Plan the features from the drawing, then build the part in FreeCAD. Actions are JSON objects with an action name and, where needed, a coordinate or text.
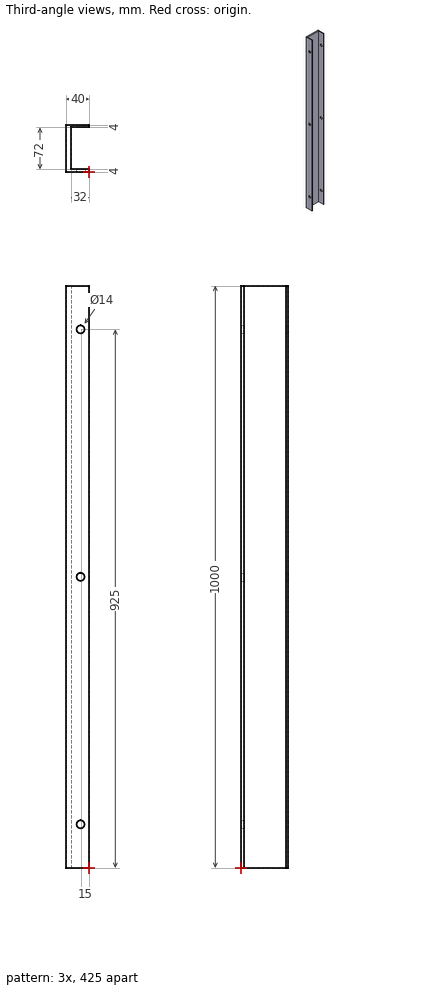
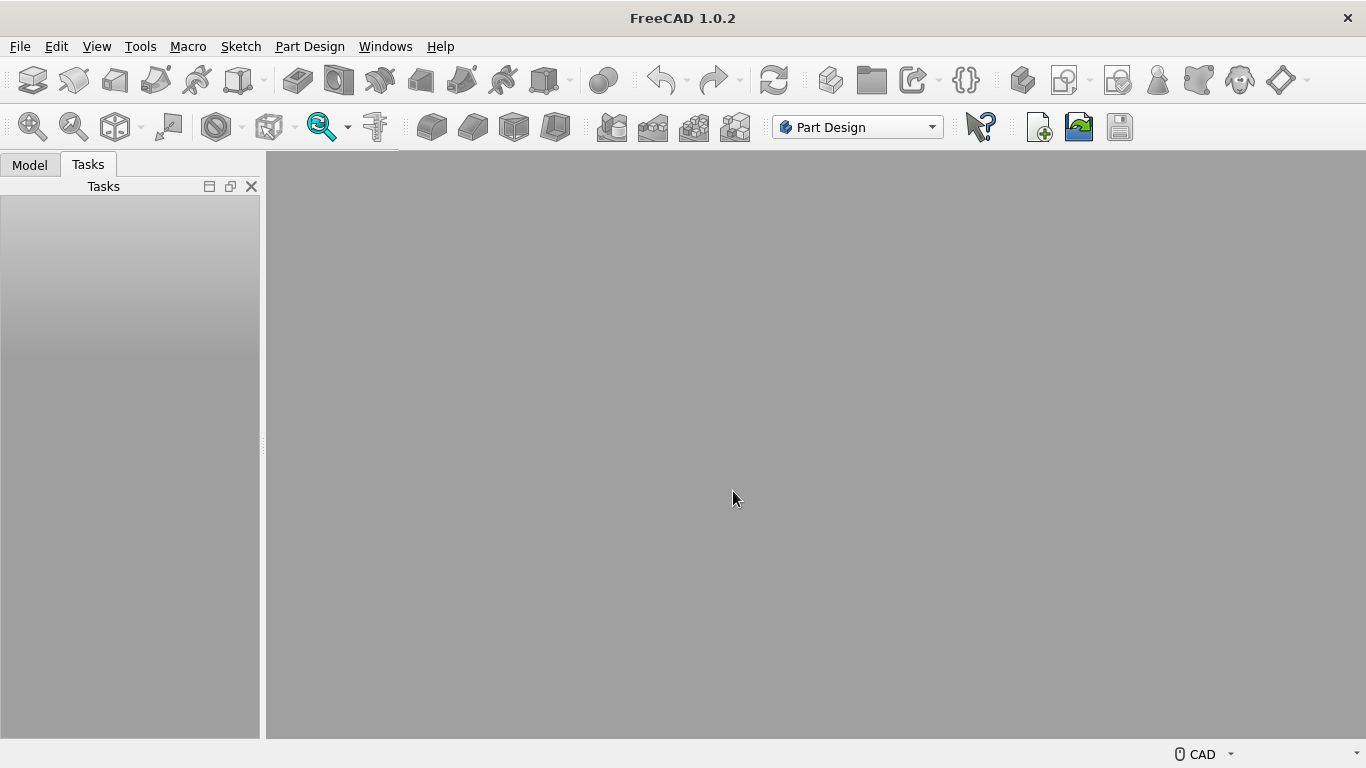
{"action": "left_click", "coordinate": [1038, 128]}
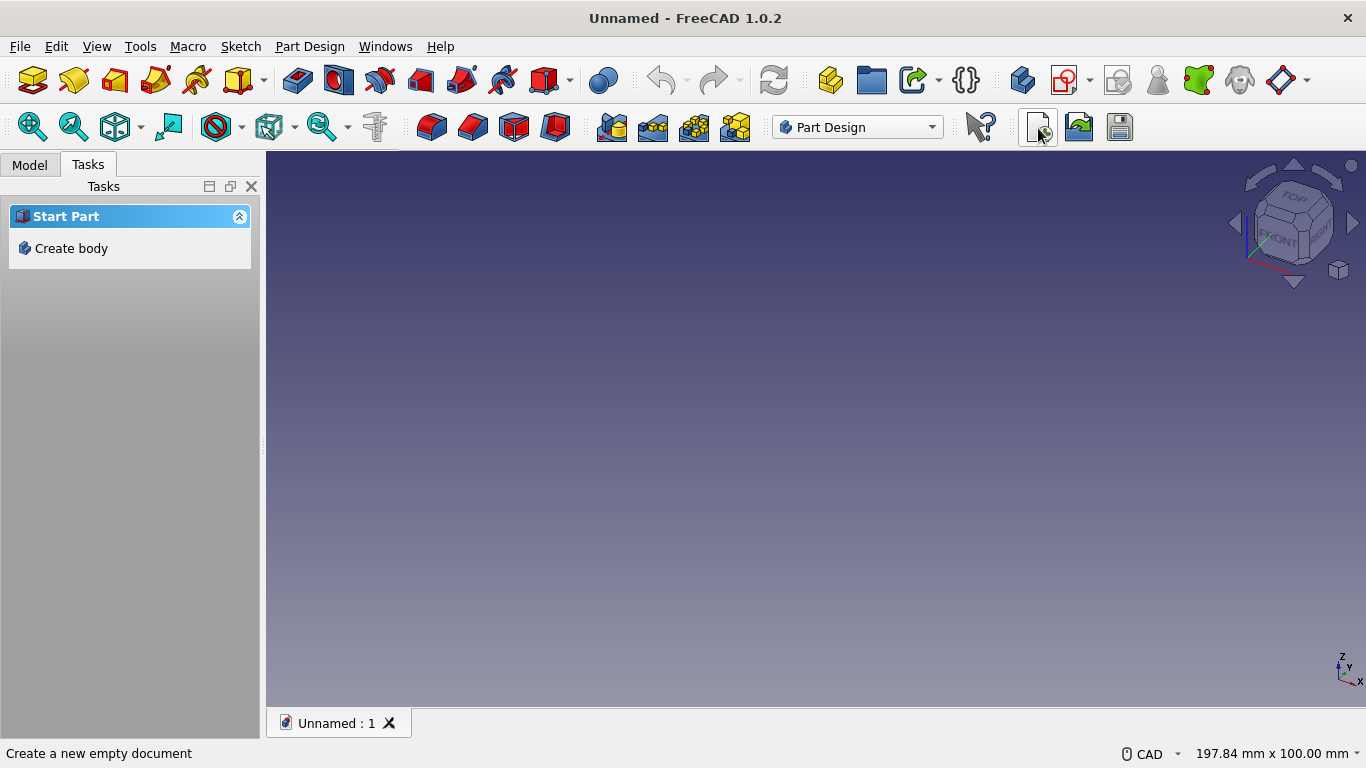
{"action": "left_click", "coordinate": [1064, 80]}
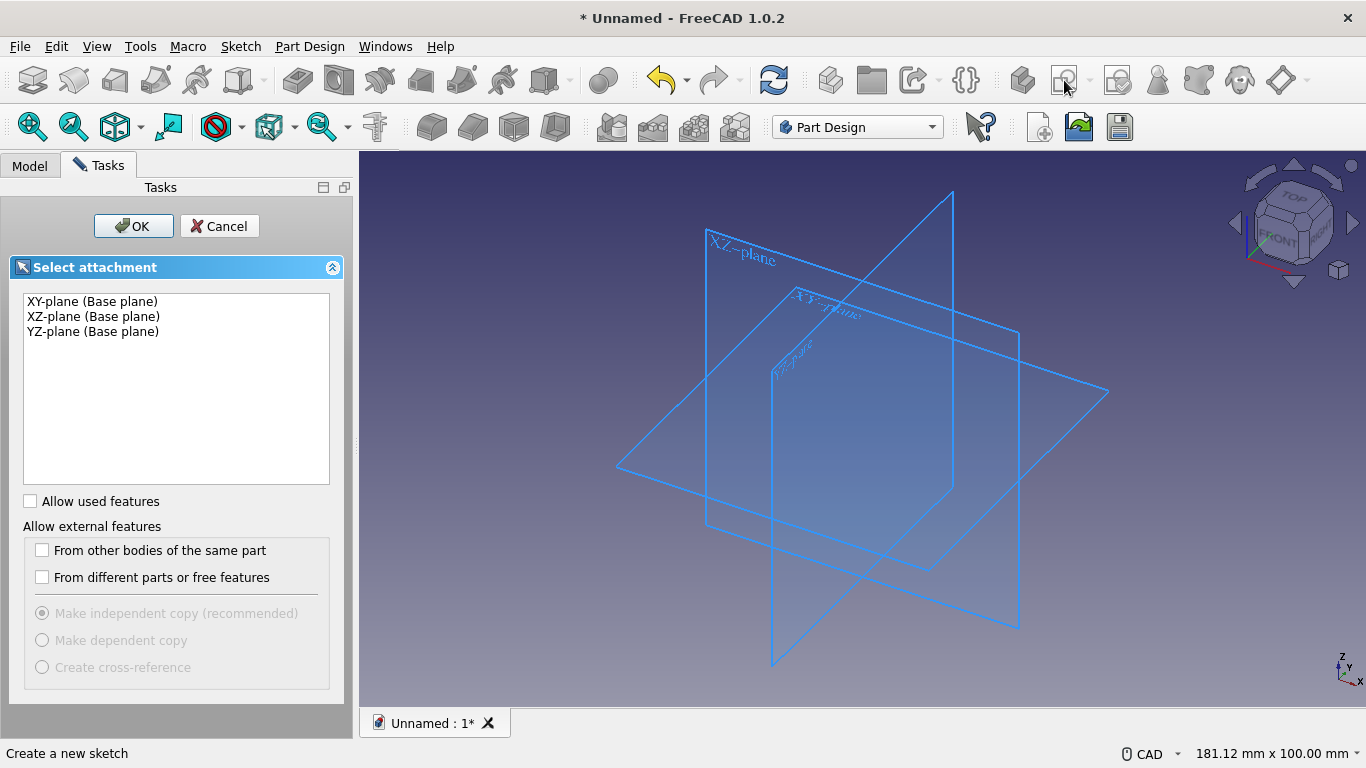
{"action": "left_click", "coordinate": [84, 302]}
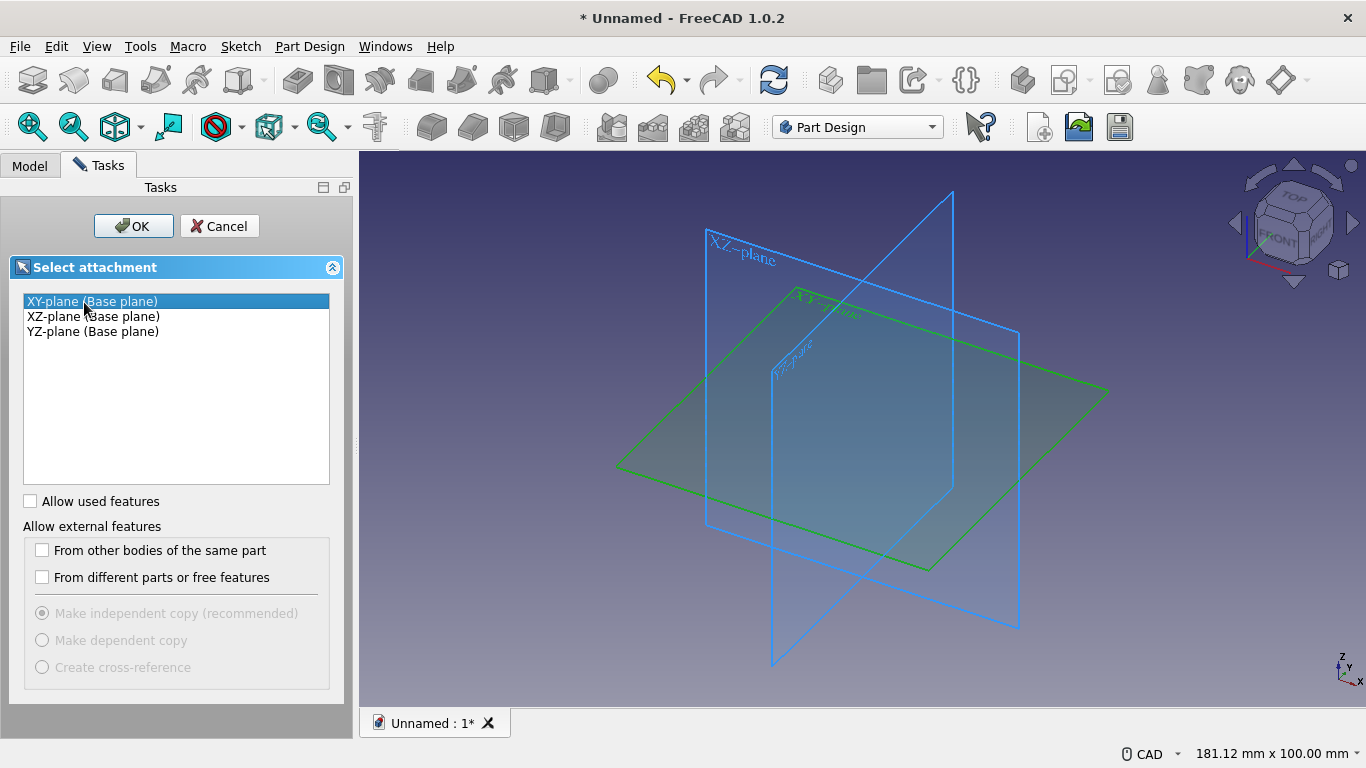
{"action": "left_click", "coordinate": [134, 226]}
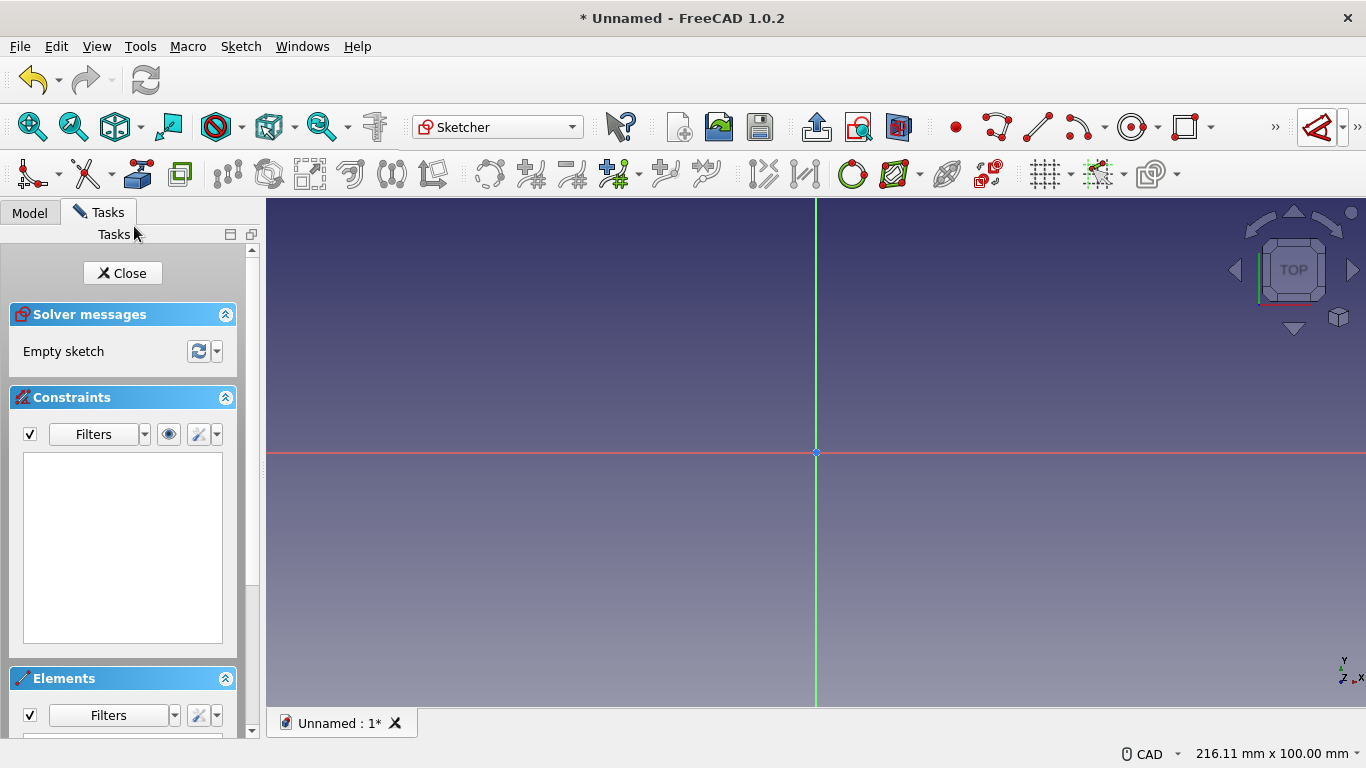
{"action": "scroll", "coordinate": [815, 679], "scroll_direction": "down", "scroll_amount": 2}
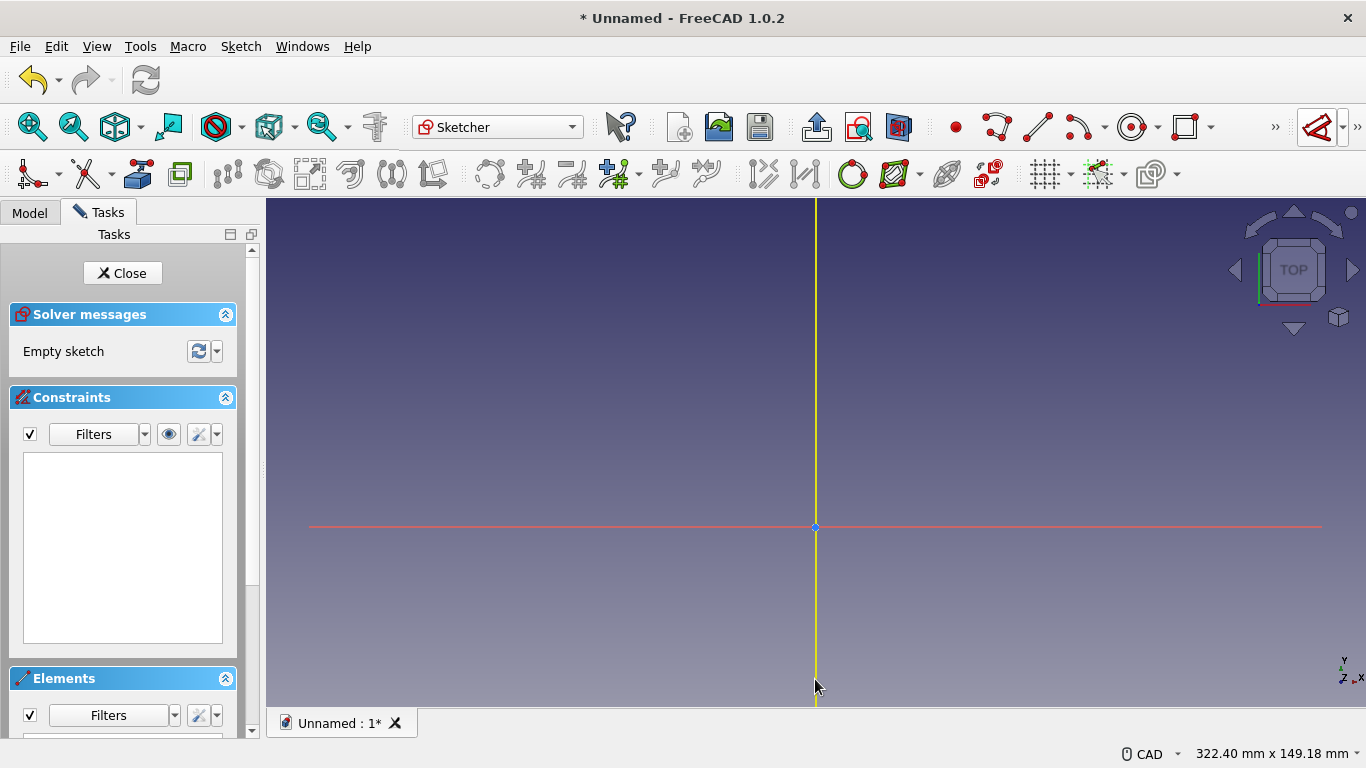
{"action": "left_click", "coordinate": [997, 128]}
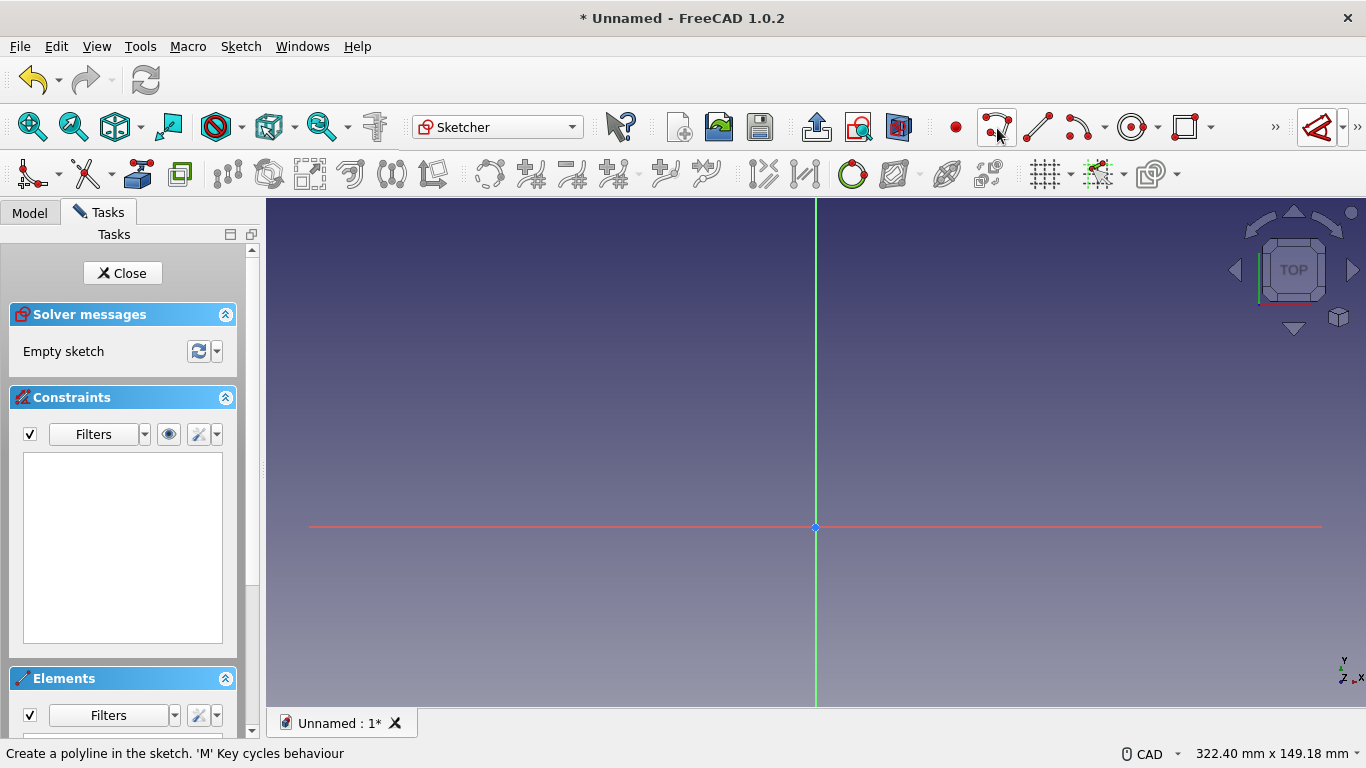
{"action": "left_click", "coordinate": [816, 527]}
{"action": "left_click", "coordinate": [807, 514]}
{"action": "left_click", "coordinate": [707, 514]}
{"action": "left_click", "coordinate": [707, 268]}
{"action": "left_click", "coordinate": [816, 268]}
{"action": "left_click", "coordinate": [807, 255]}
{"action": "left_click", "coordinate": [679, 255]}
{"action": "left_click", "coordinate": [679, 518]}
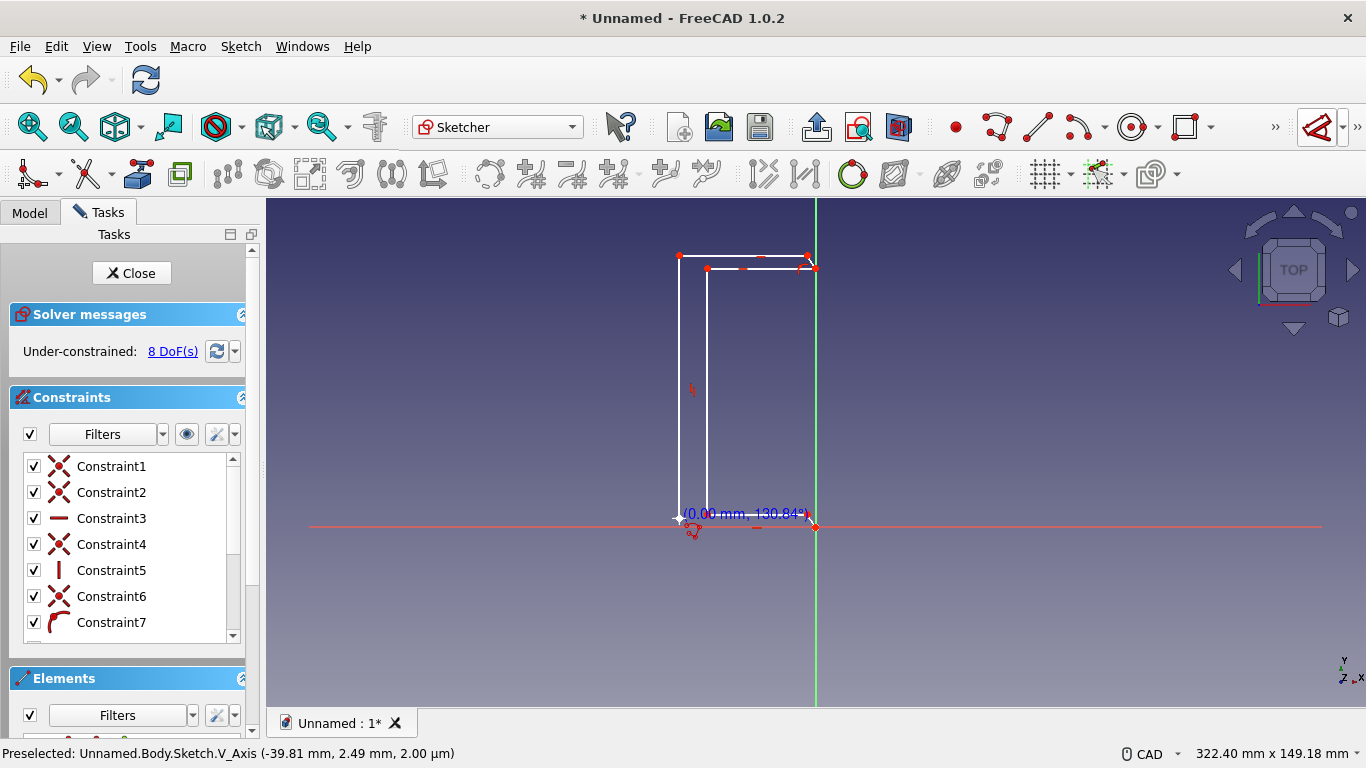
{"action": "scroll", "coordinate": [816, 527], "scroll_direction": "up", "scroll_amount": 5}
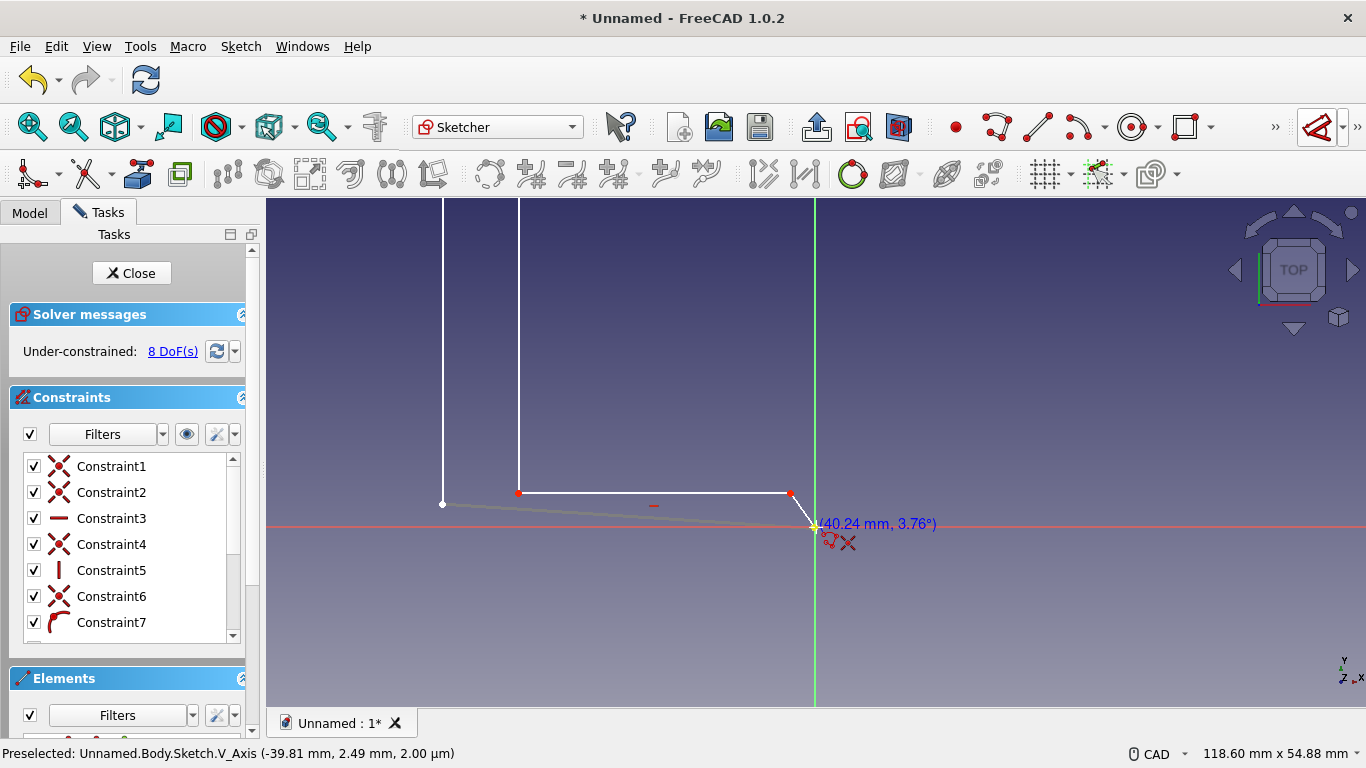
{"action": "left_click", "coordinate": [815, 527]}
{"action": "key", "text": "Escape"}
{"action": "key", "text": "Escape"}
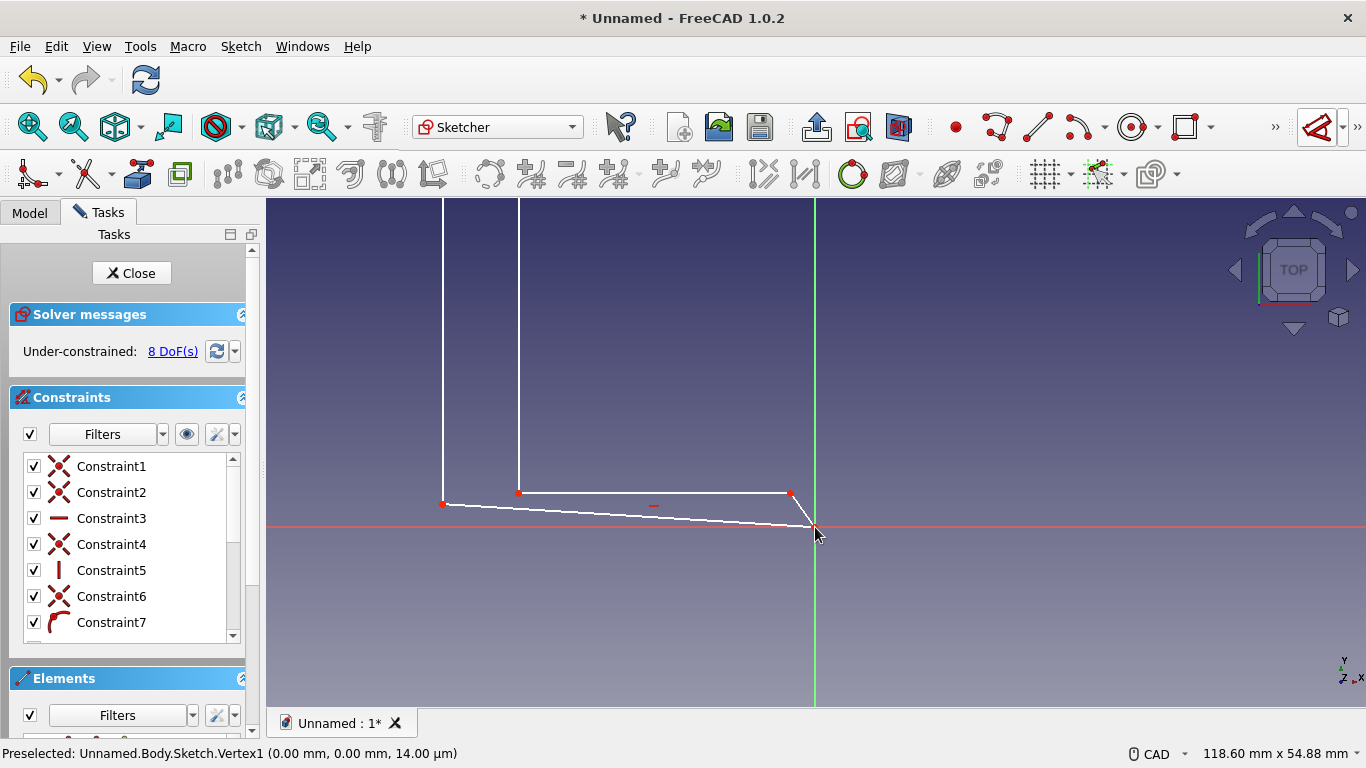
{"action": "left_click", "coordinate": [798, 503]}